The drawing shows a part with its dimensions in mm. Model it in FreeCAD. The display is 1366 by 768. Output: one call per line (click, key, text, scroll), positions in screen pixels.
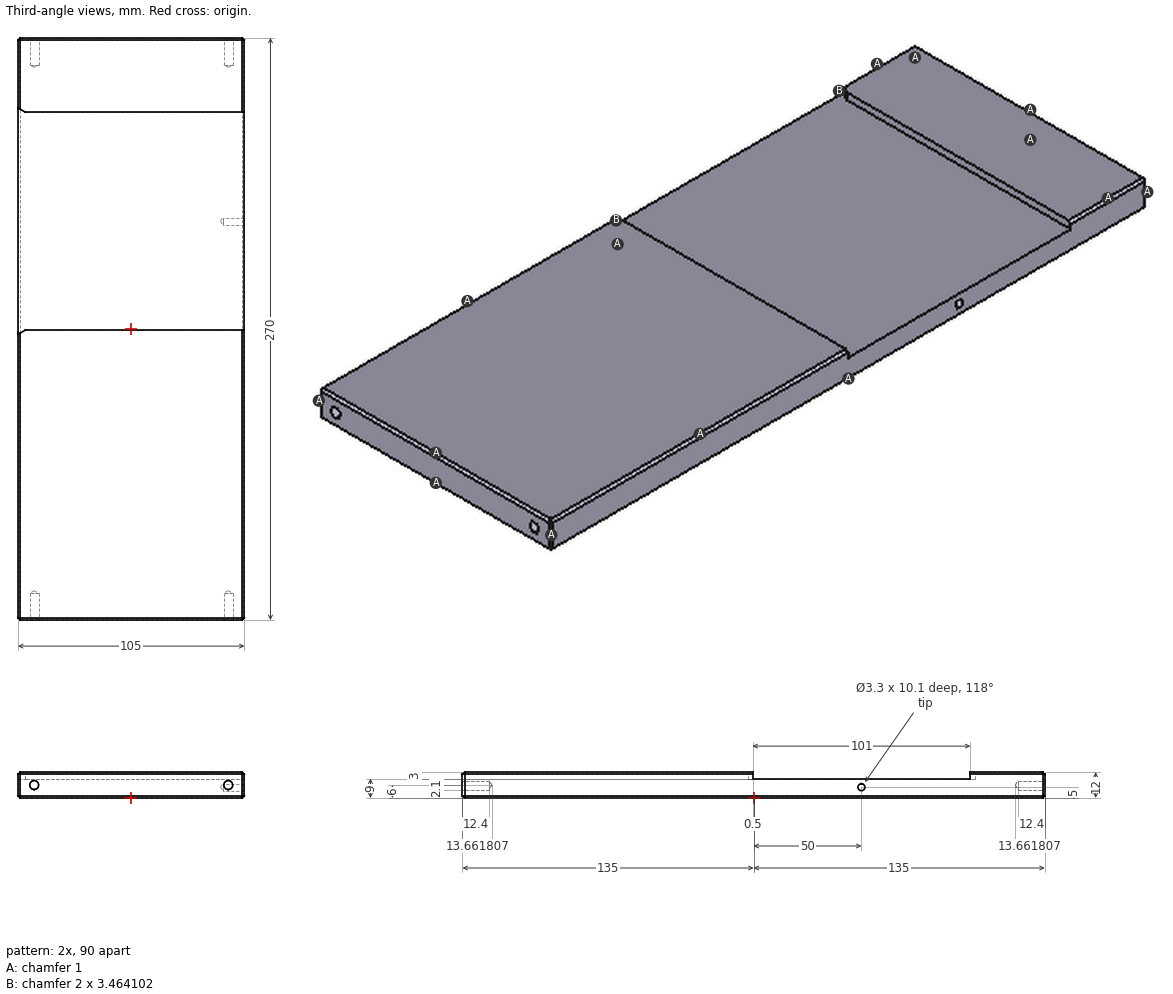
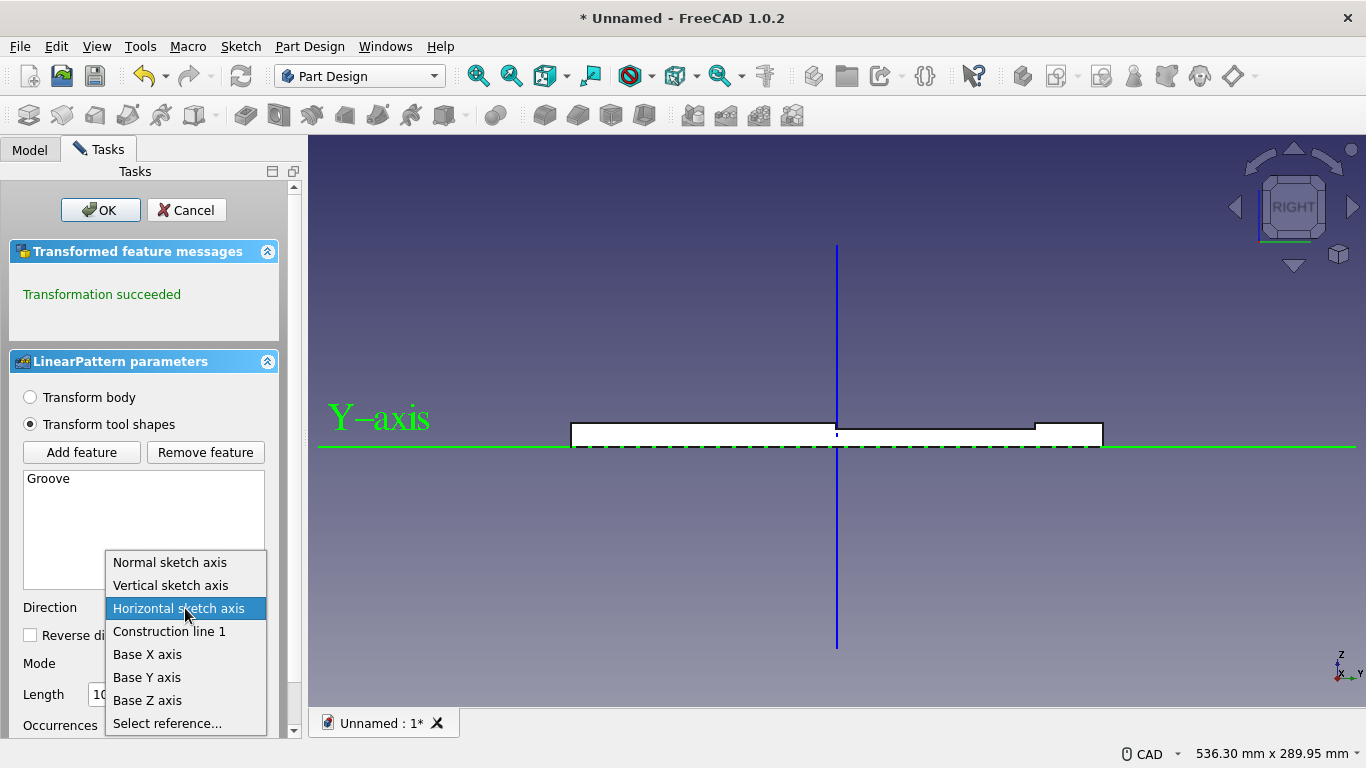
click(184, 654)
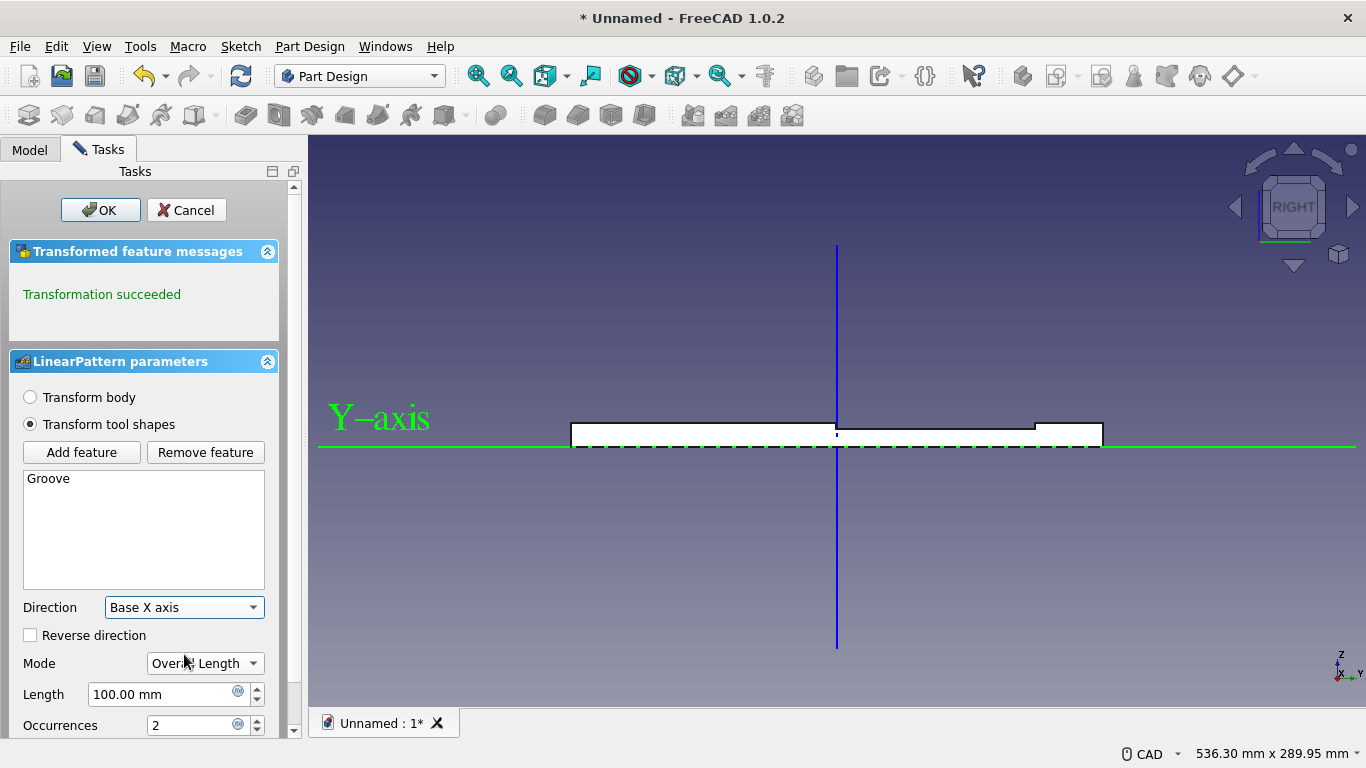
click(206, 664)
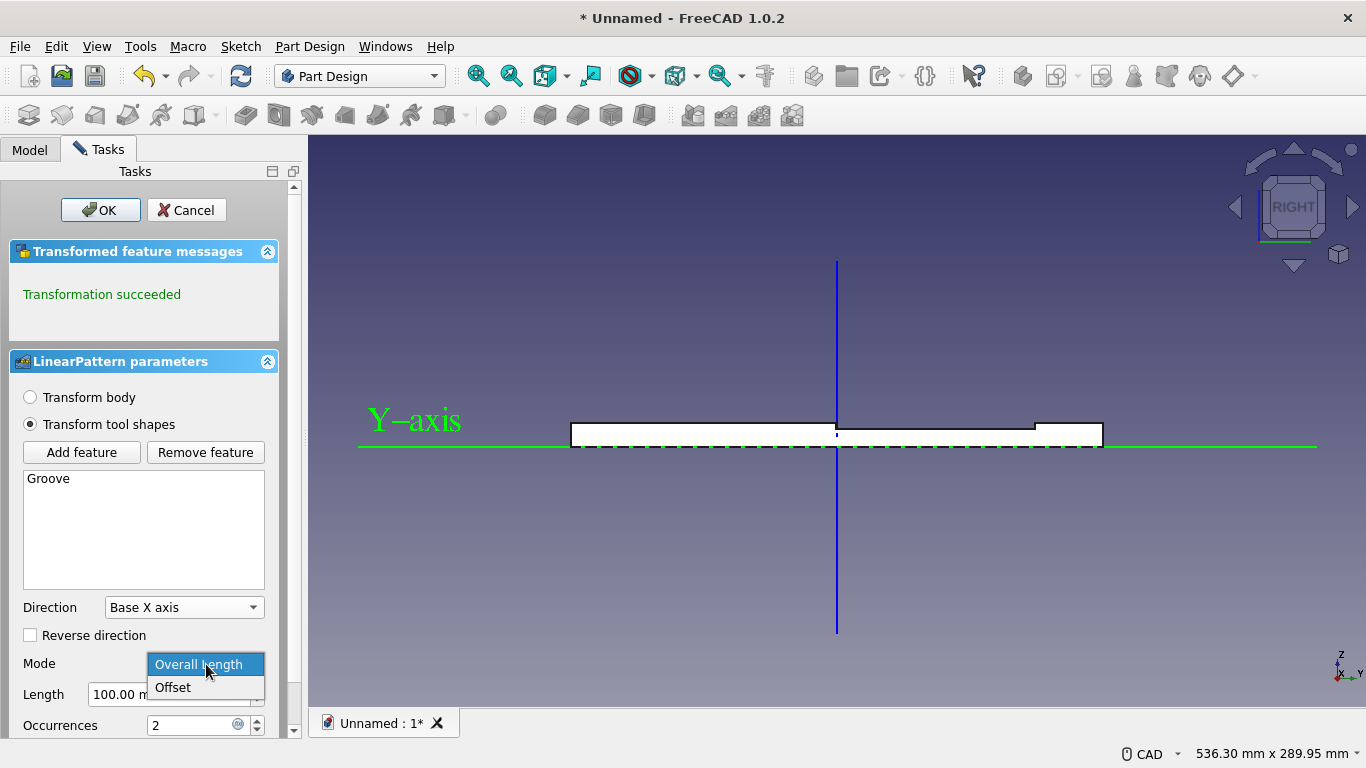
click(204, 688)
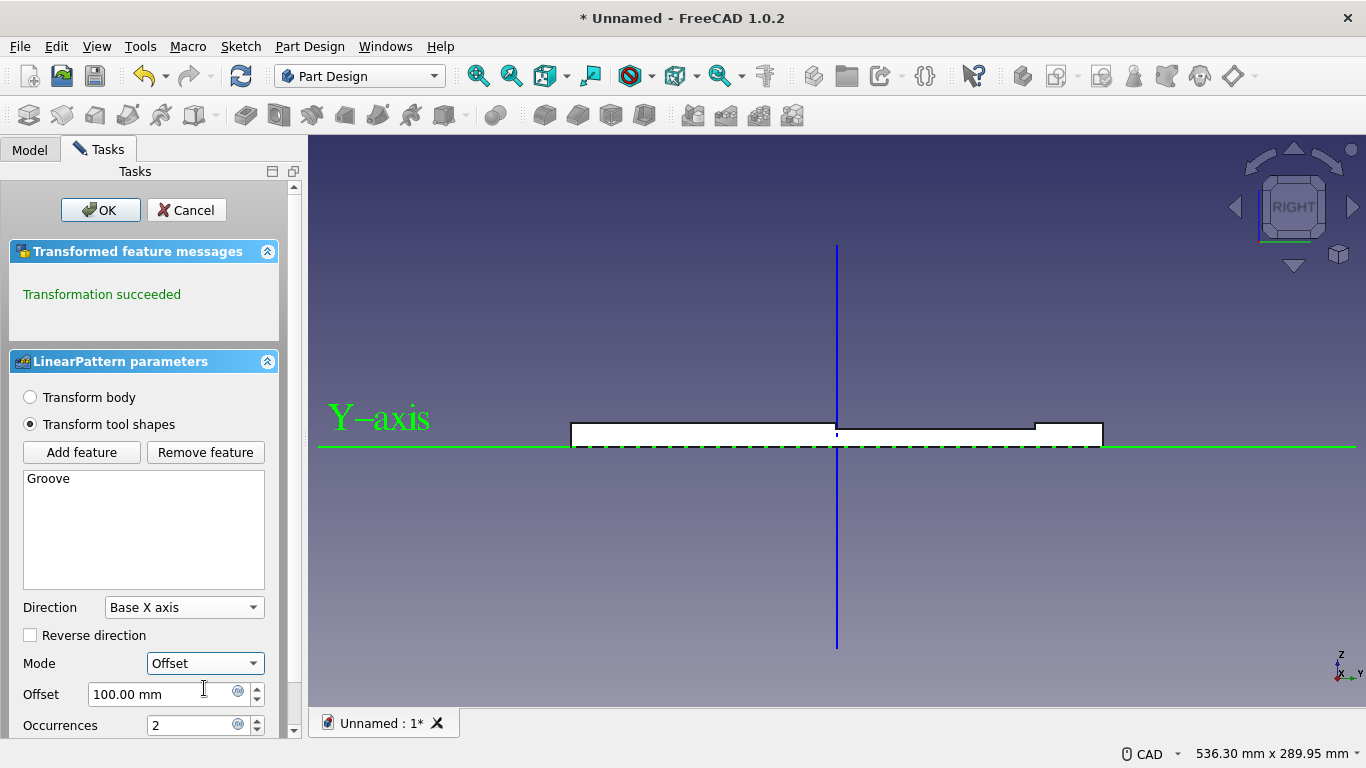
triple_click(170, 694)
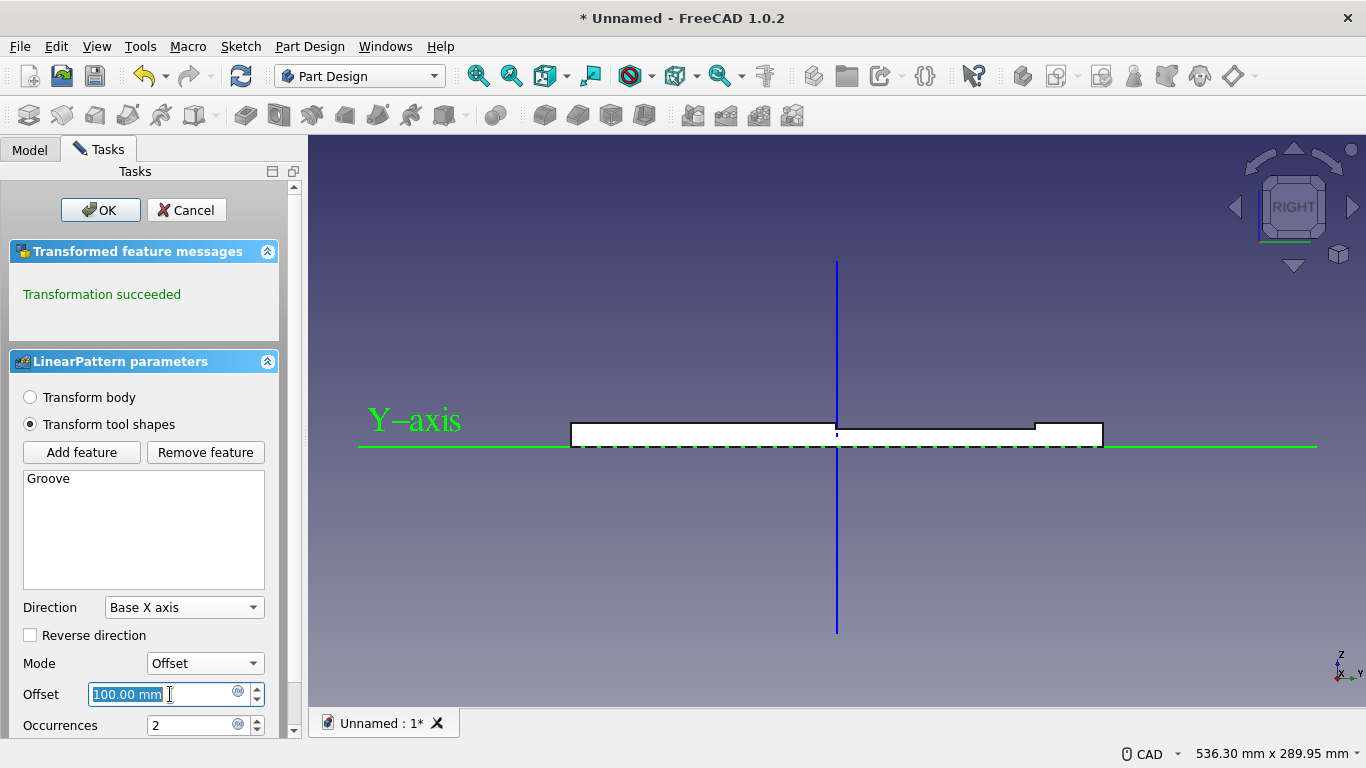
text(90)
key(Tab)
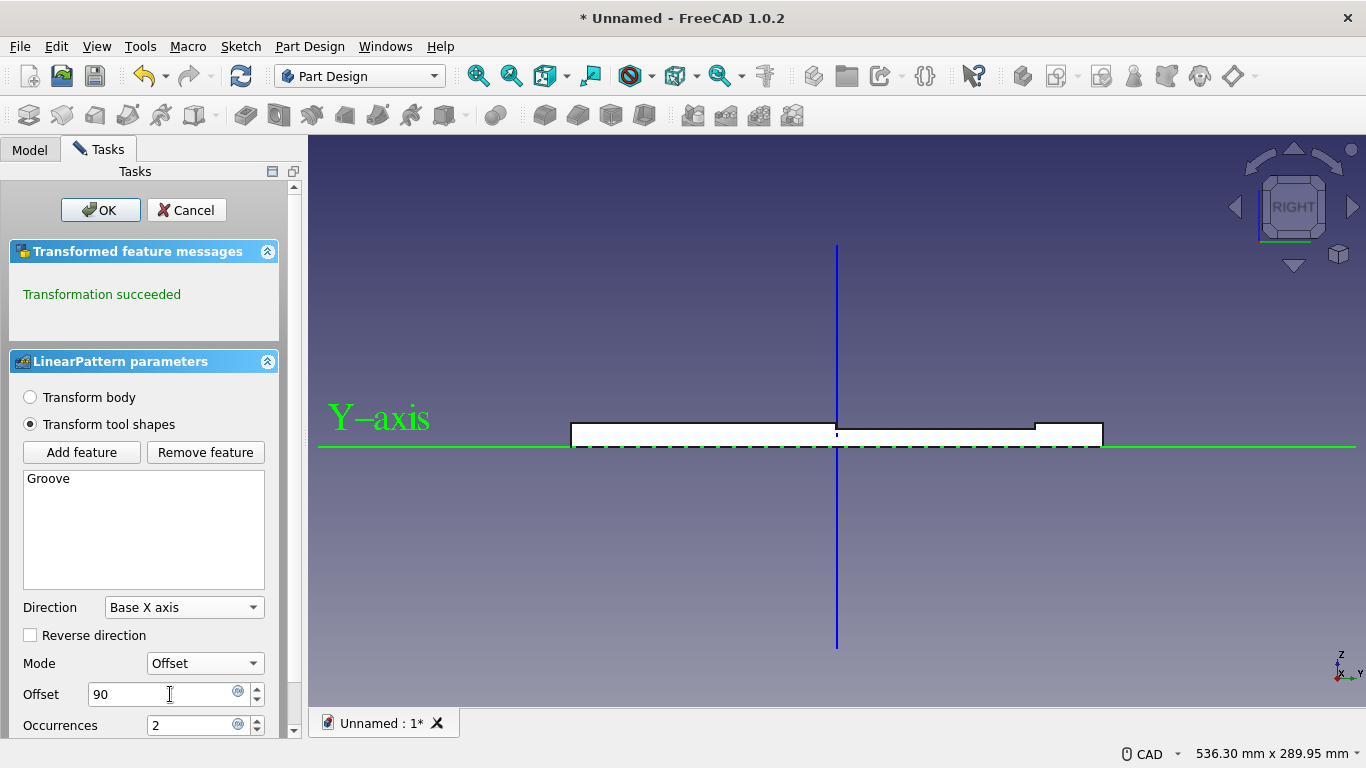
triple_click(199, 726)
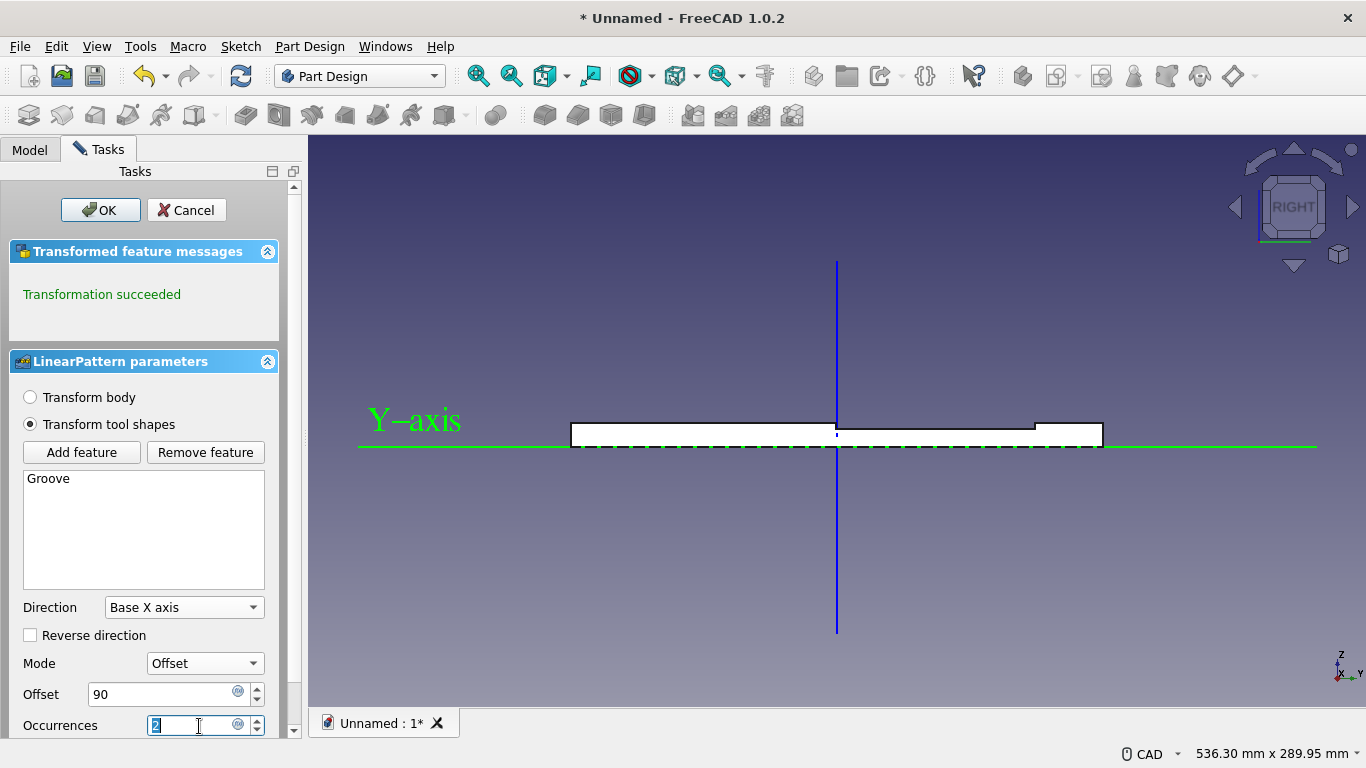
text(2)
key(Tab)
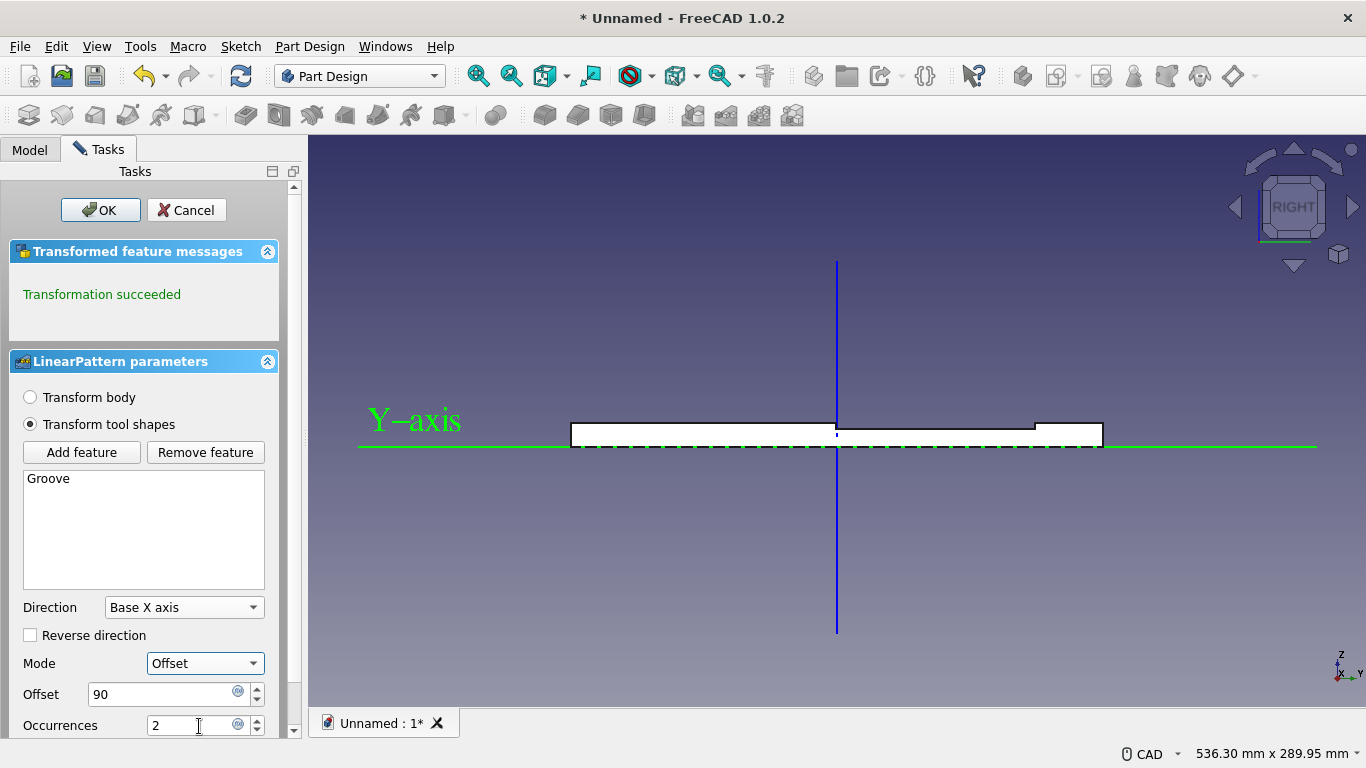
click(101, 210)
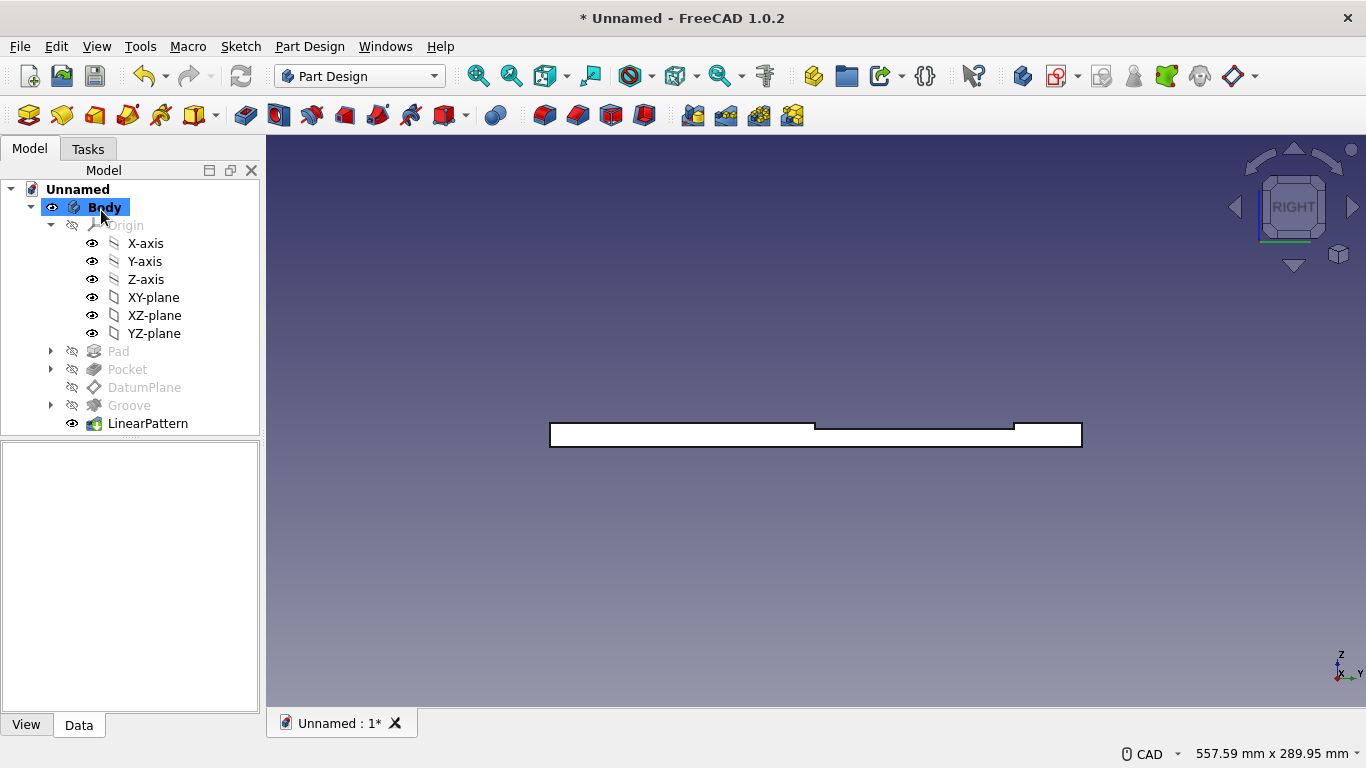
click(117, 405)